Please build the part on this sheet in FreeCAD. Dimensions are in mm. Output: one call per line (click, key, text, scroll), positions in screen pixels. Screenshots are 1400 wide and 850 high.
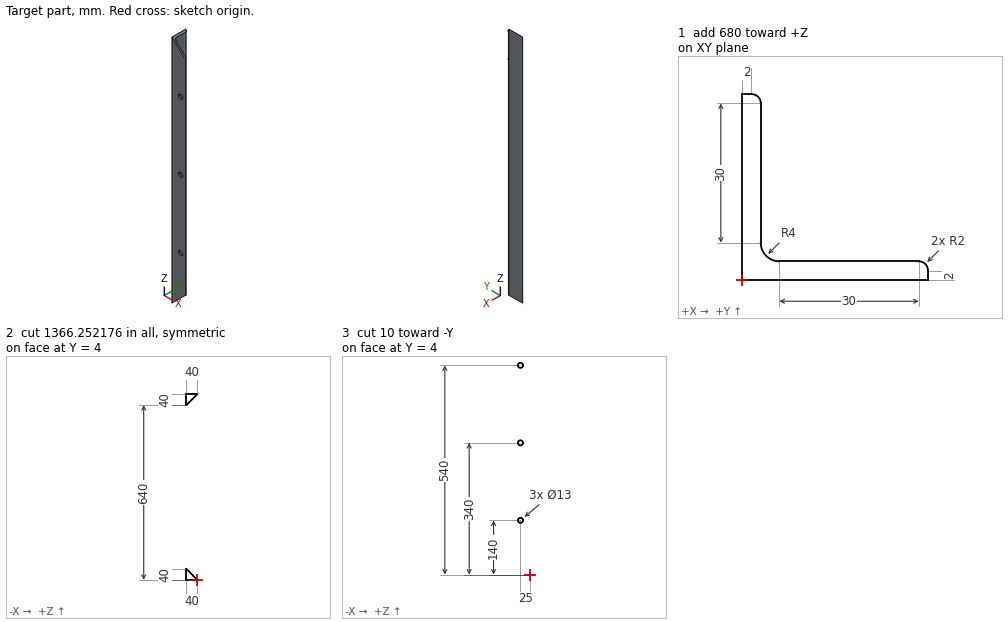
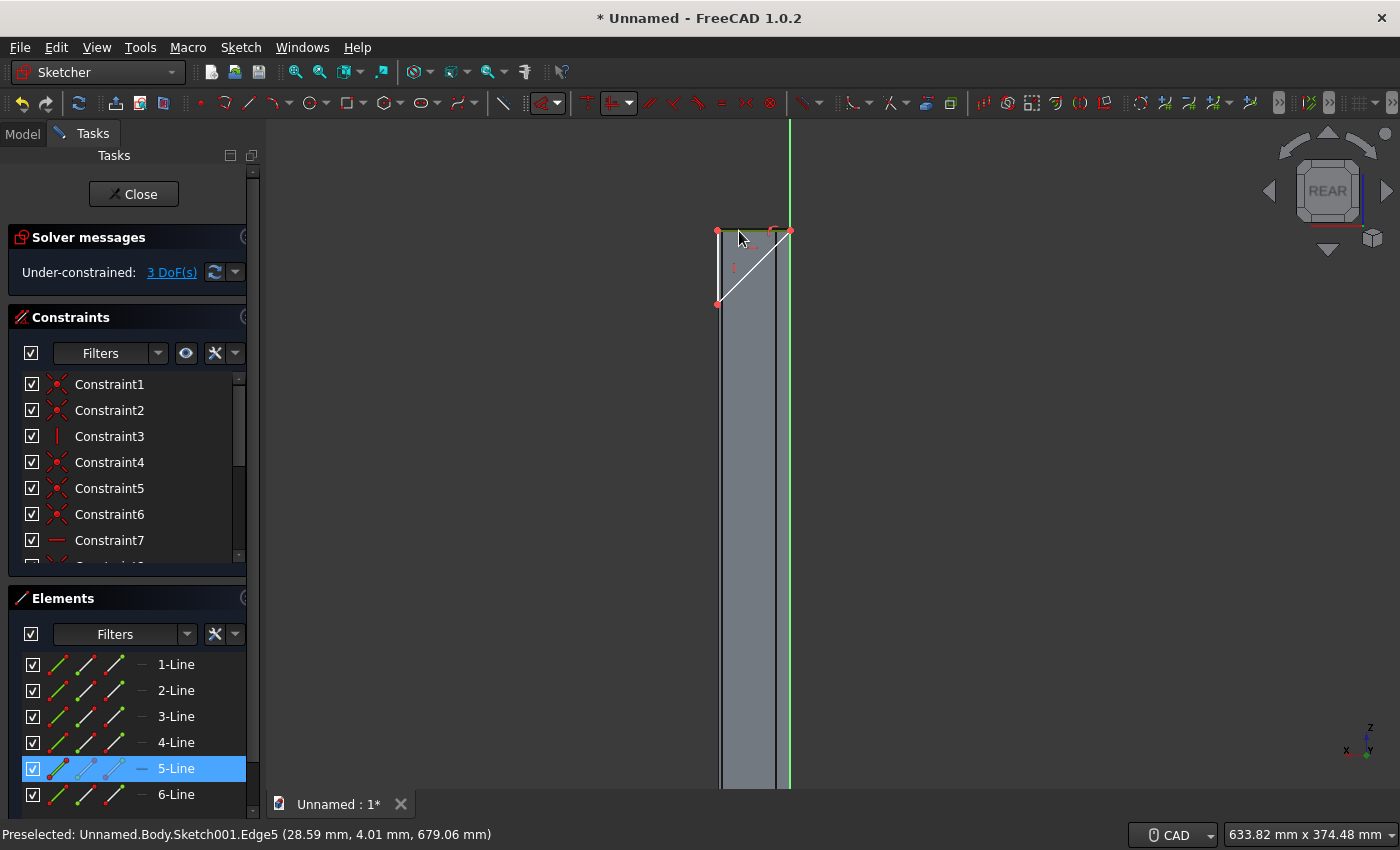
key(l)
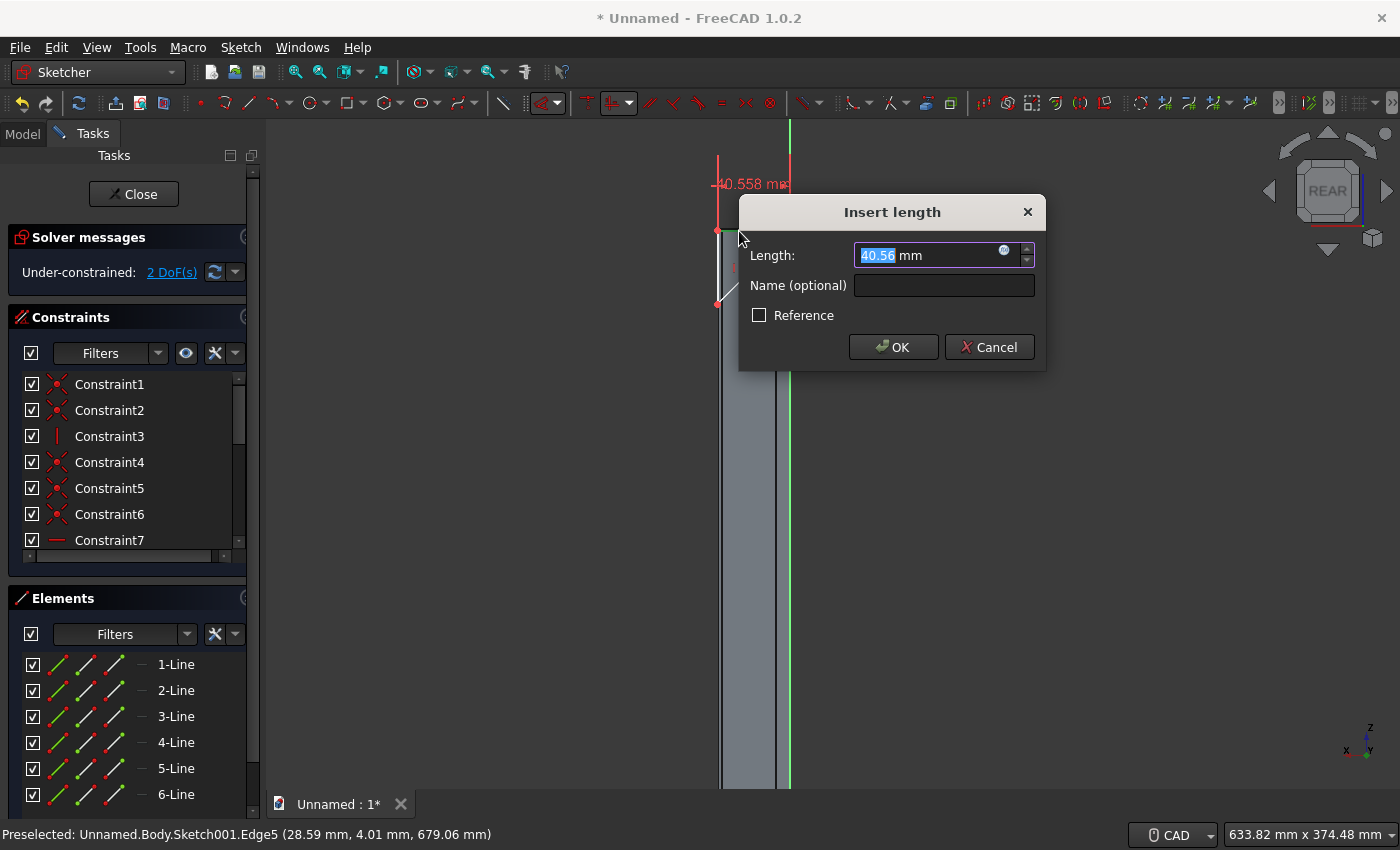
text(40)
key(Return)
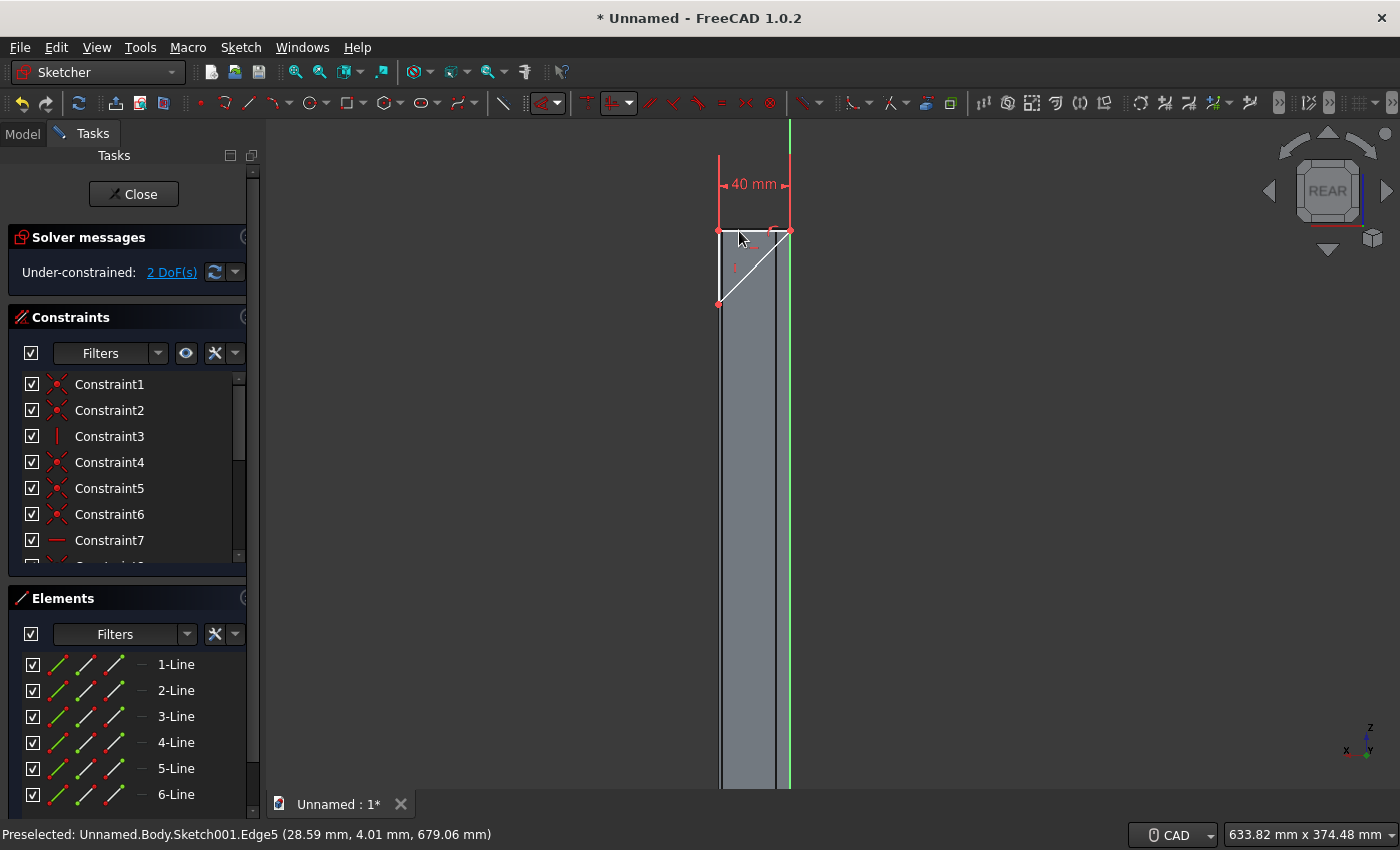
click(719, 253)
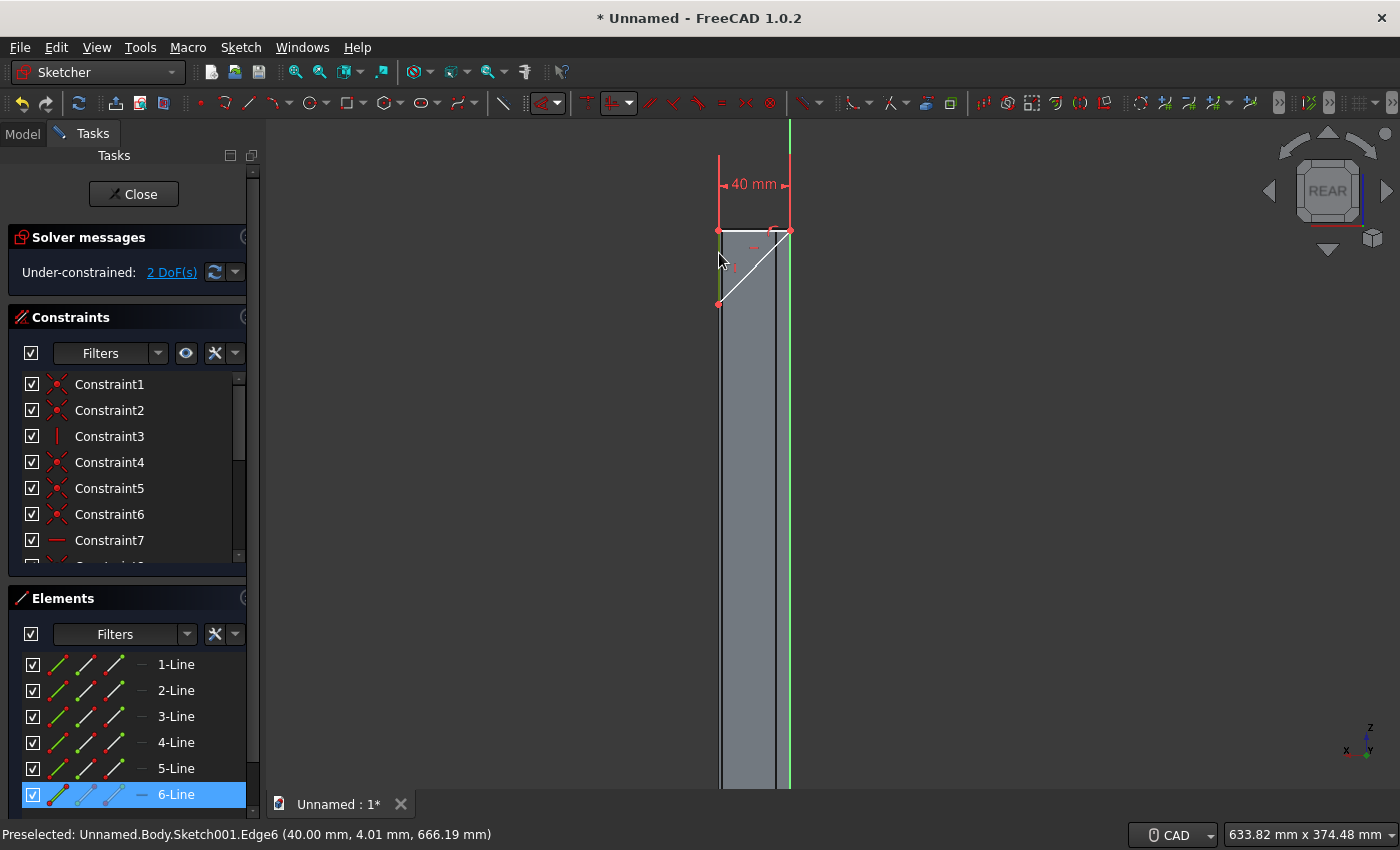
click(560, 104)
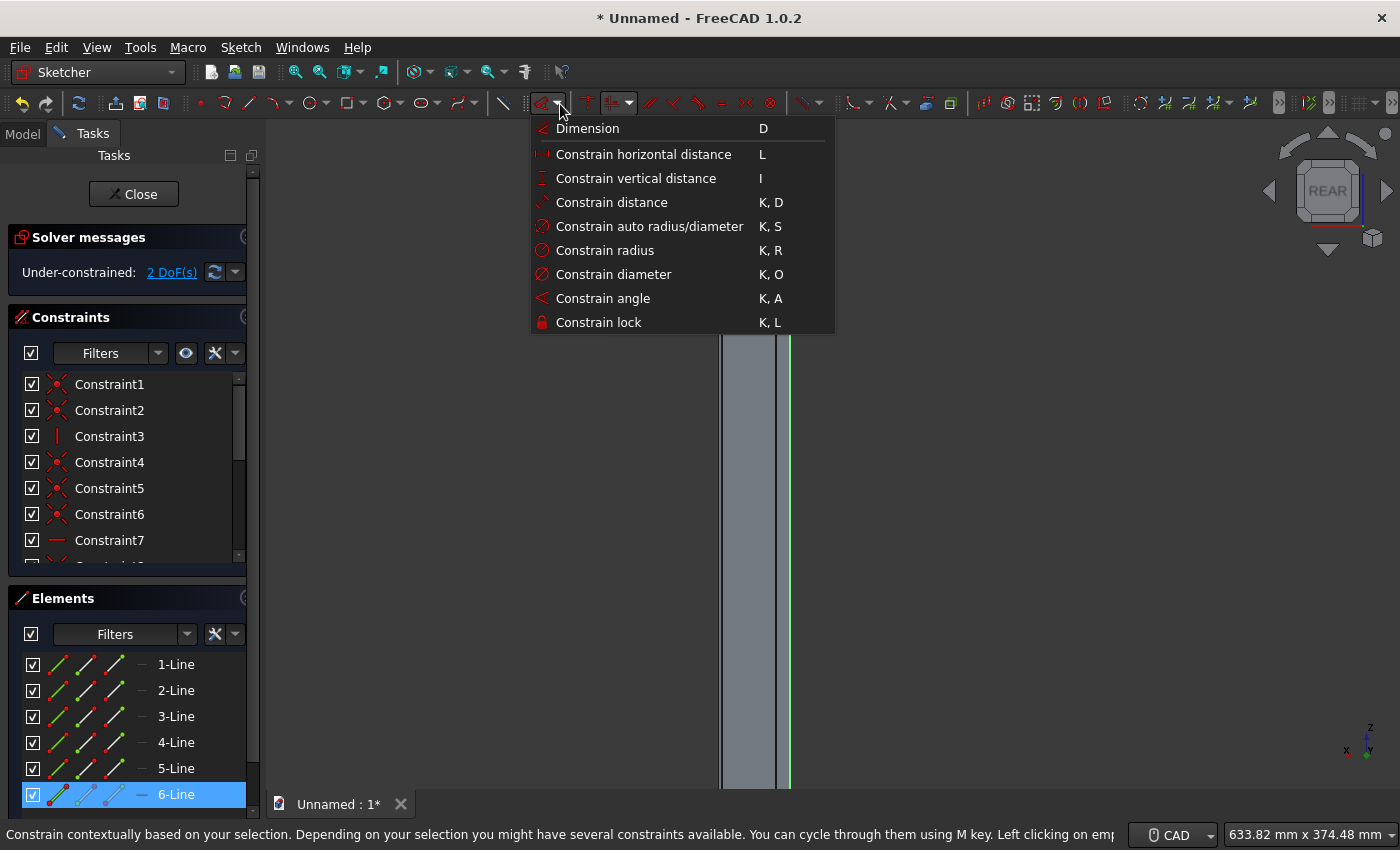
click(683, 178)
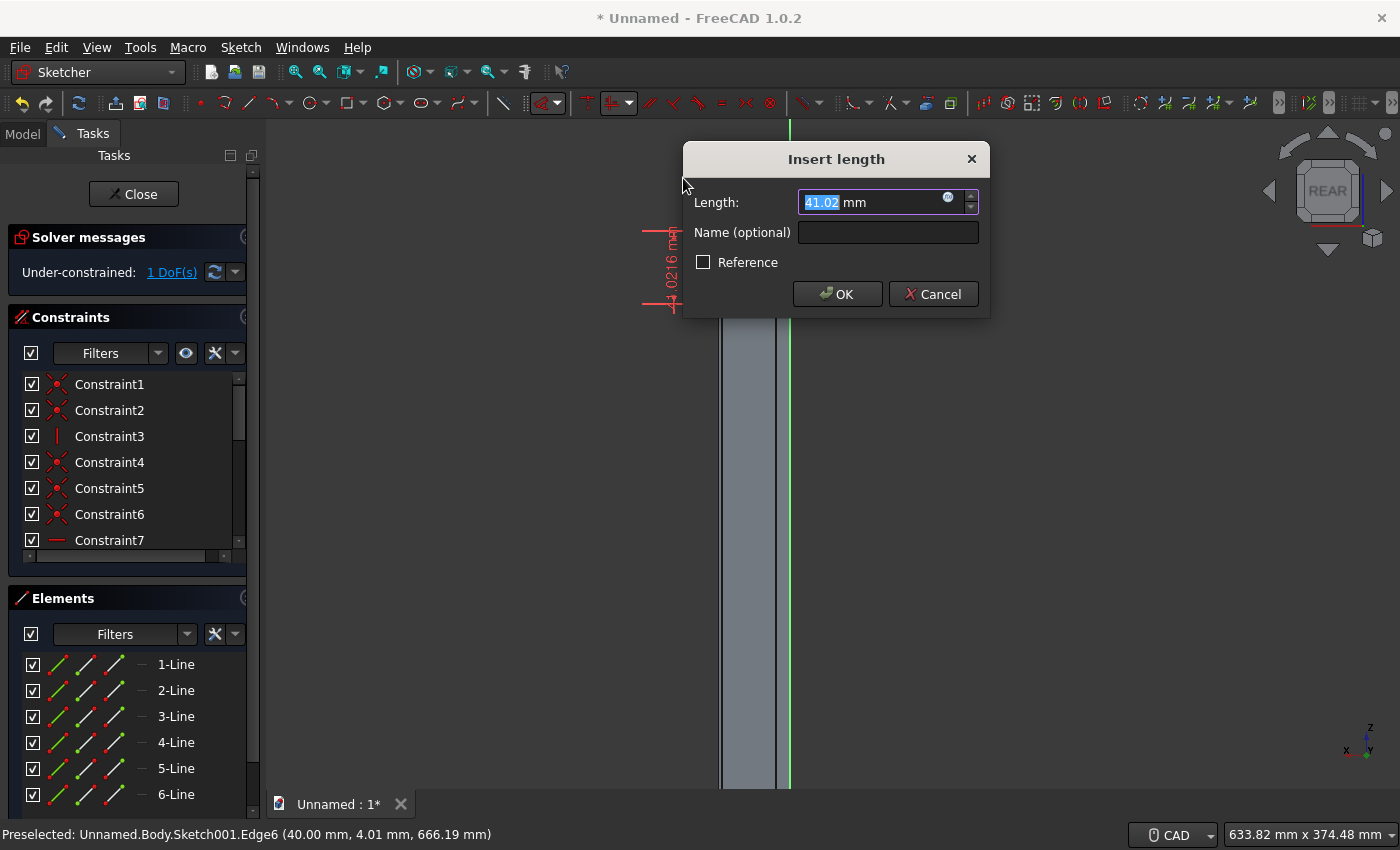
text(40)
key(Return)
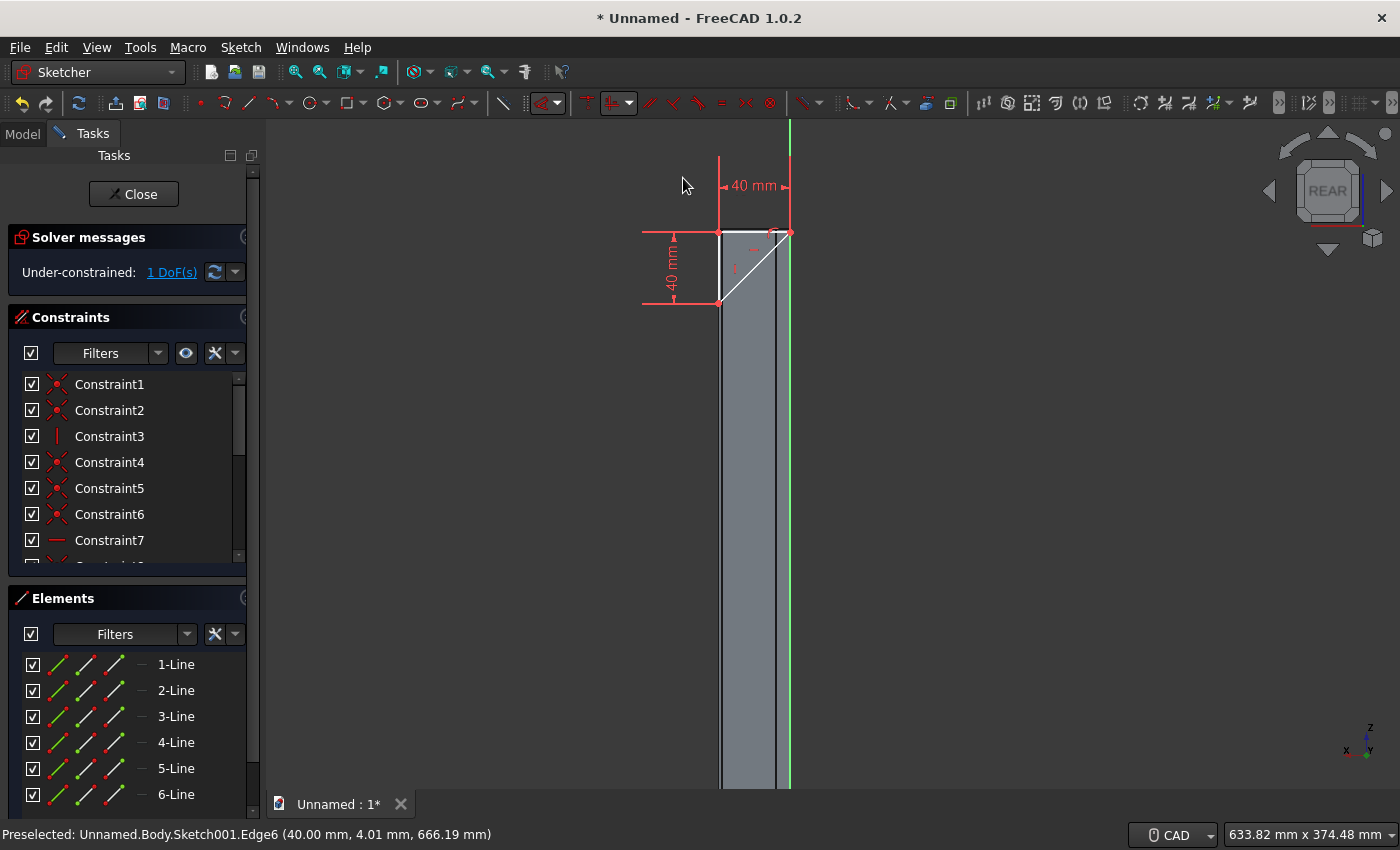
click(719, 304)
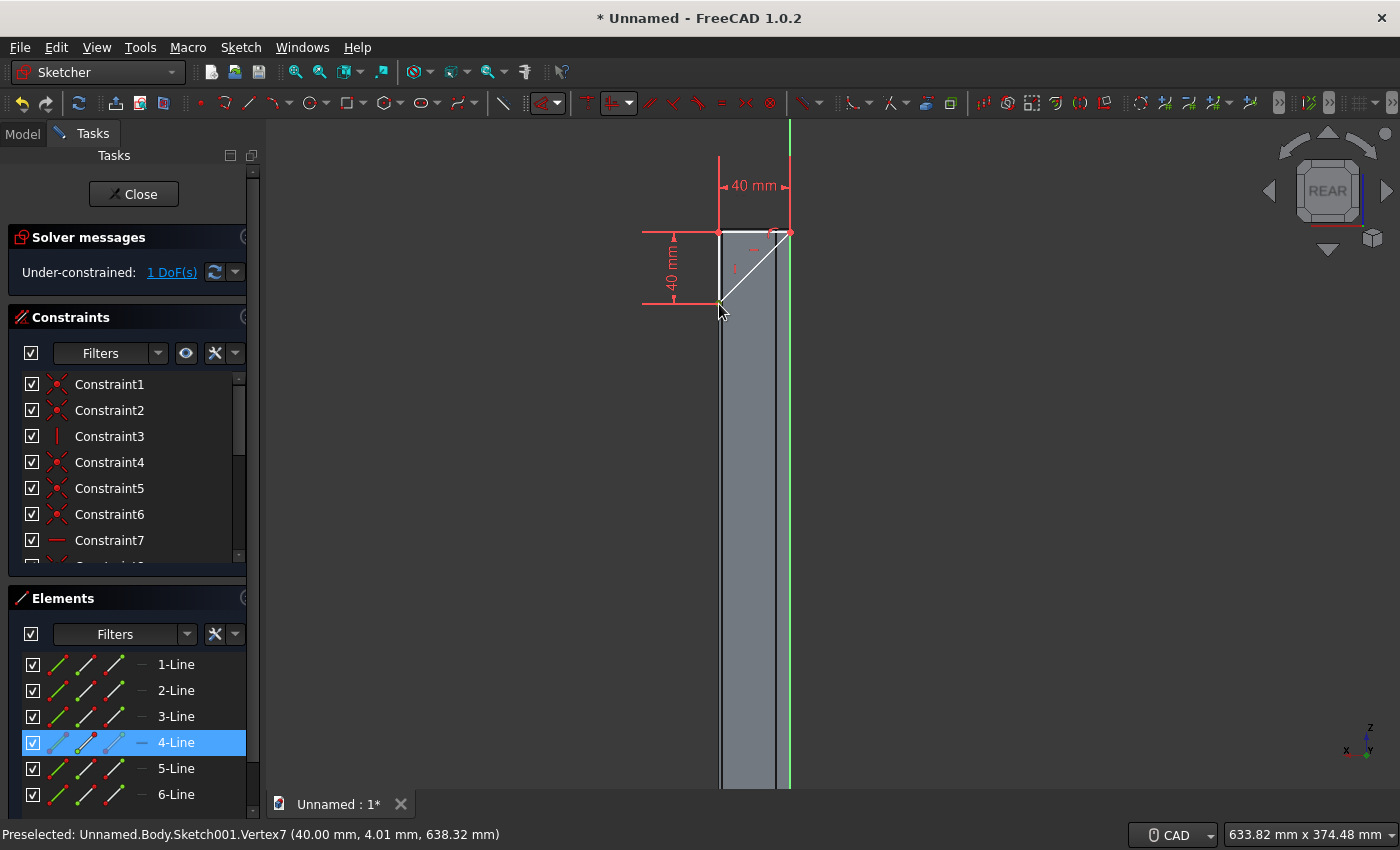
click(560, 104)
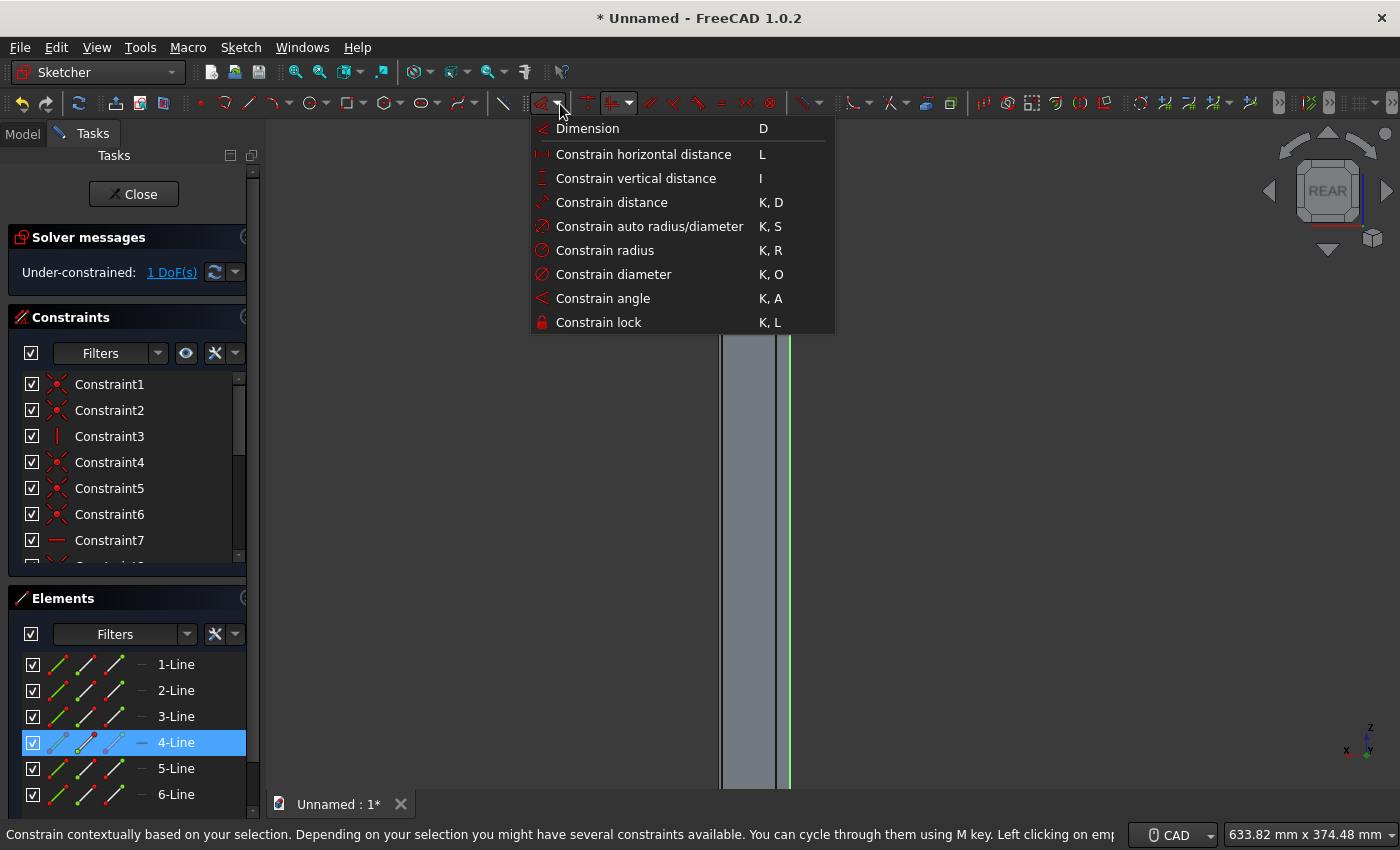
click(683, 178)